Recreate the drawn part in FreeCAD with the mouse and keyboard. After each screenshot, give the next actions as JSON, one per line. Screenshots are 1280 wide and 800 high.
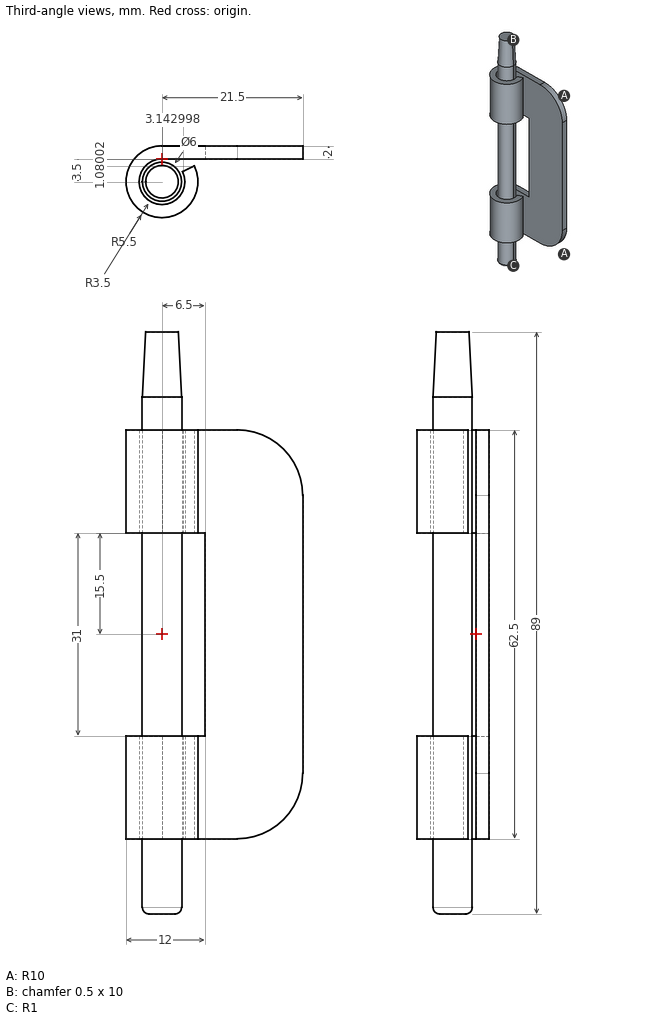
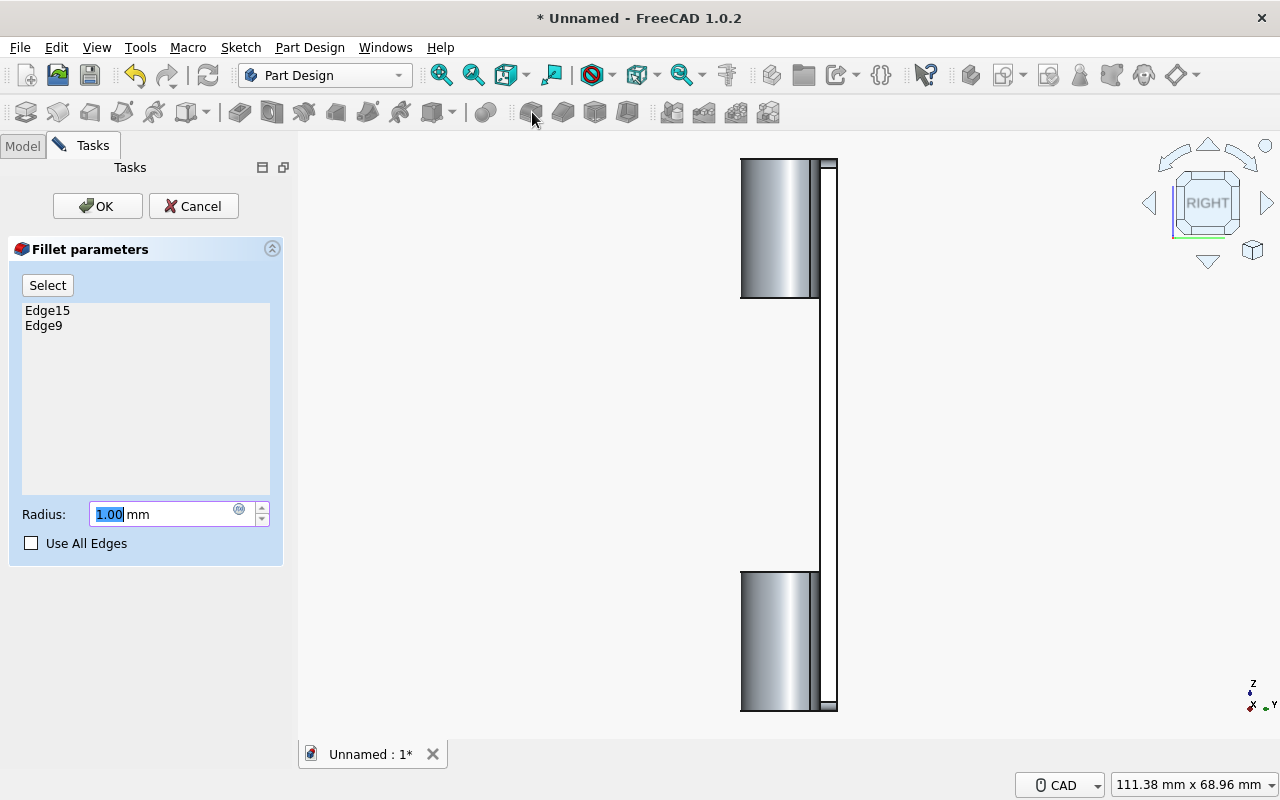
{"action": "type", "text": "10"}
{"action": "key", "text": "Tab"}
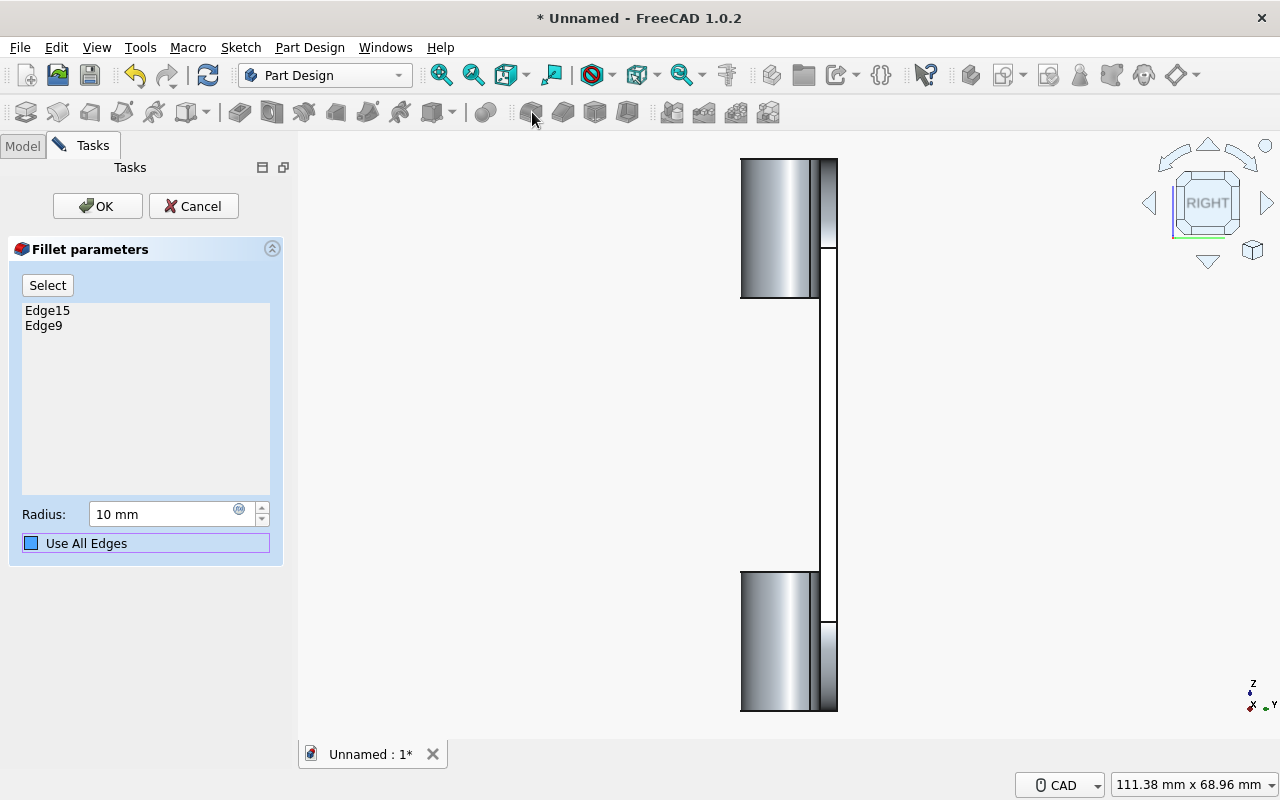
{"action": "left_click", "coordinate": [98, 206]}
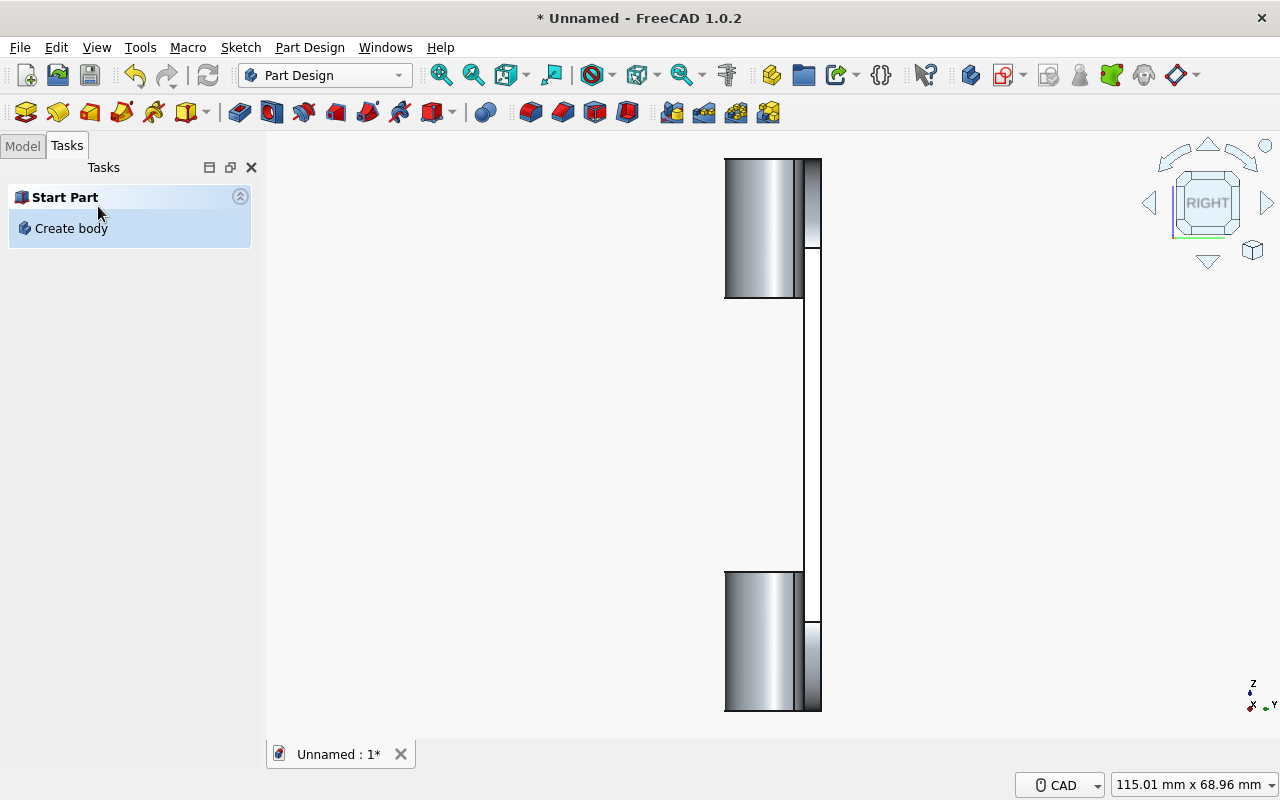
{"action": "left_click", "coordinate": [972, 76]}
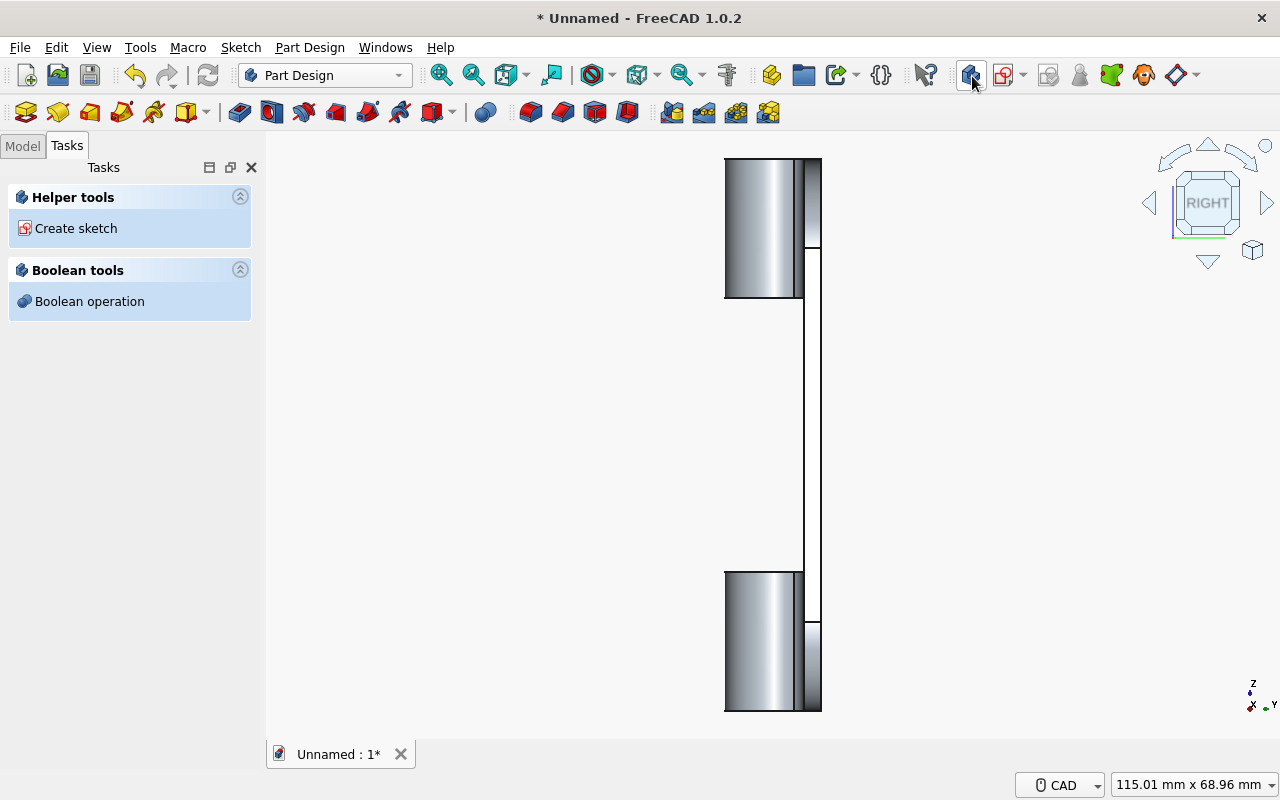
{"action": "left_click", "coordinate": [23, 145]}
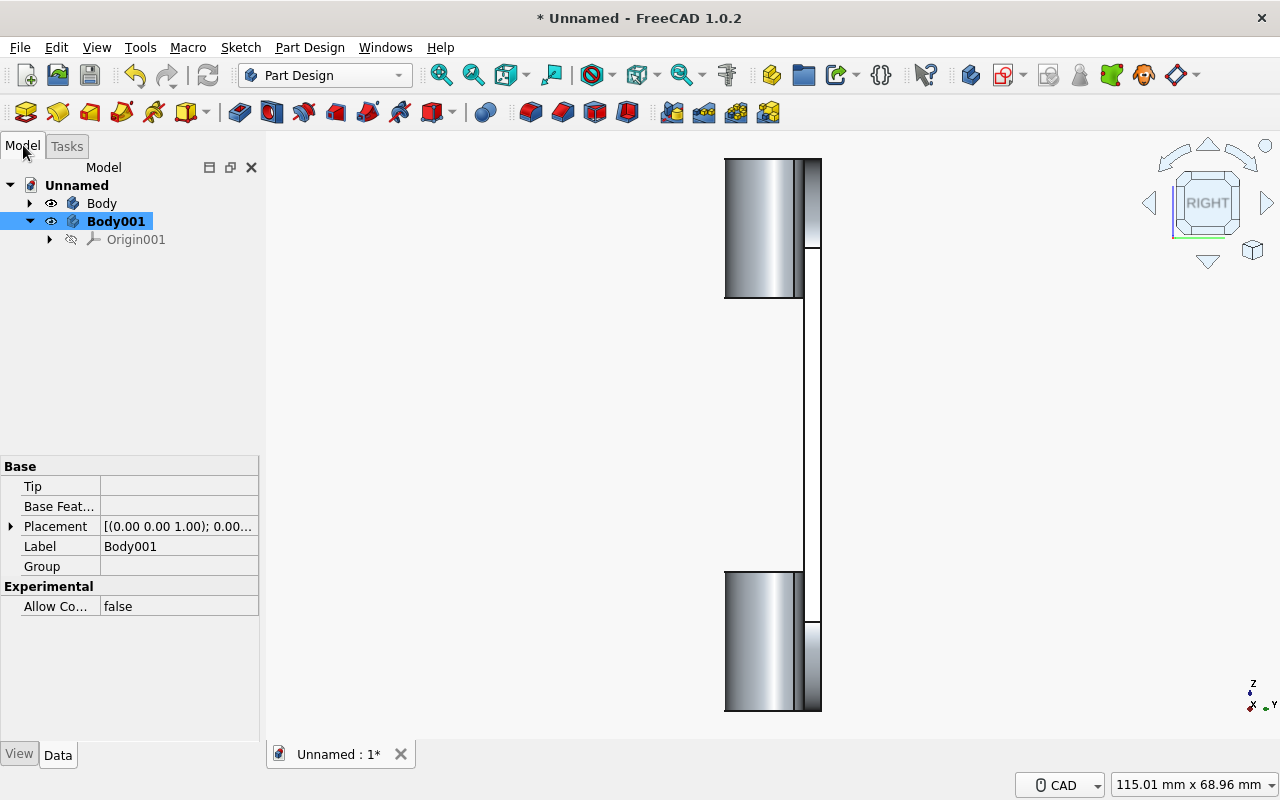
{"action": "left_click", "coordinate": [50, 239]}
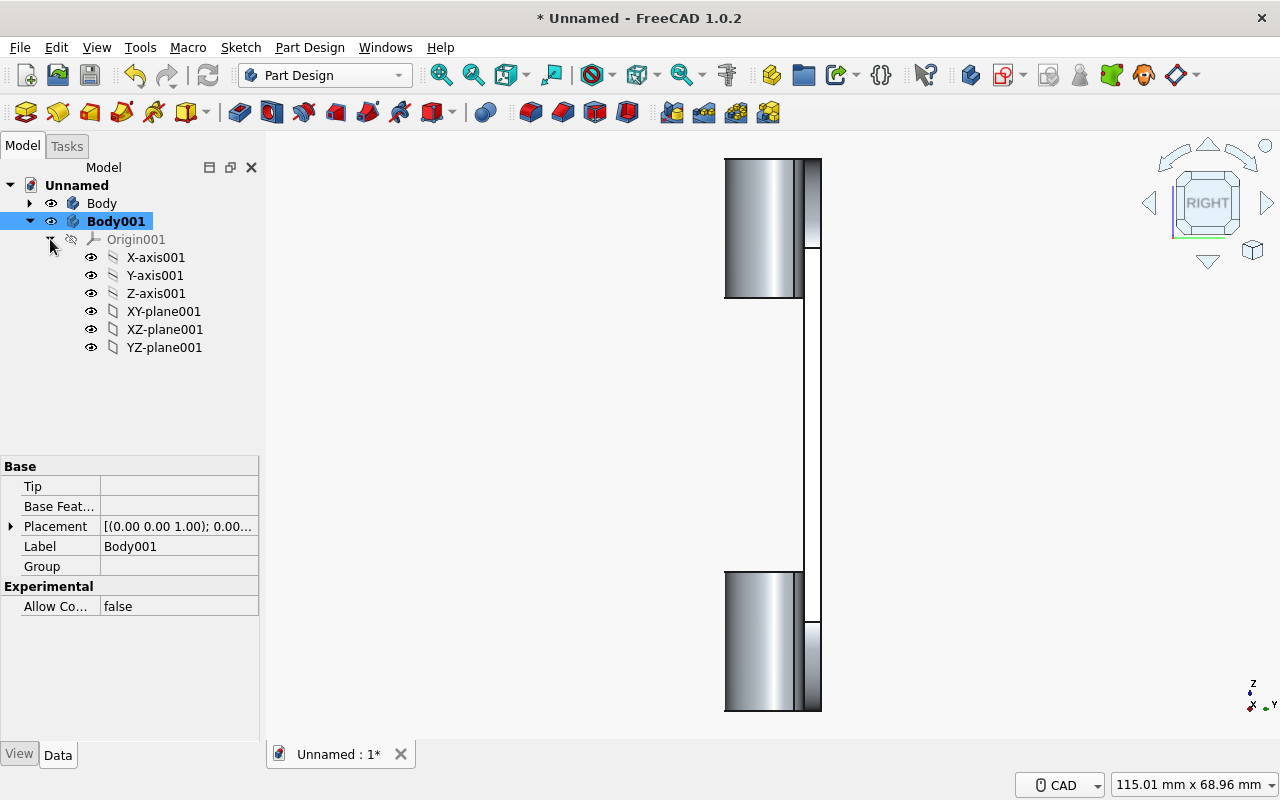
{"action": "left_click", "coordinate": [136, 311]}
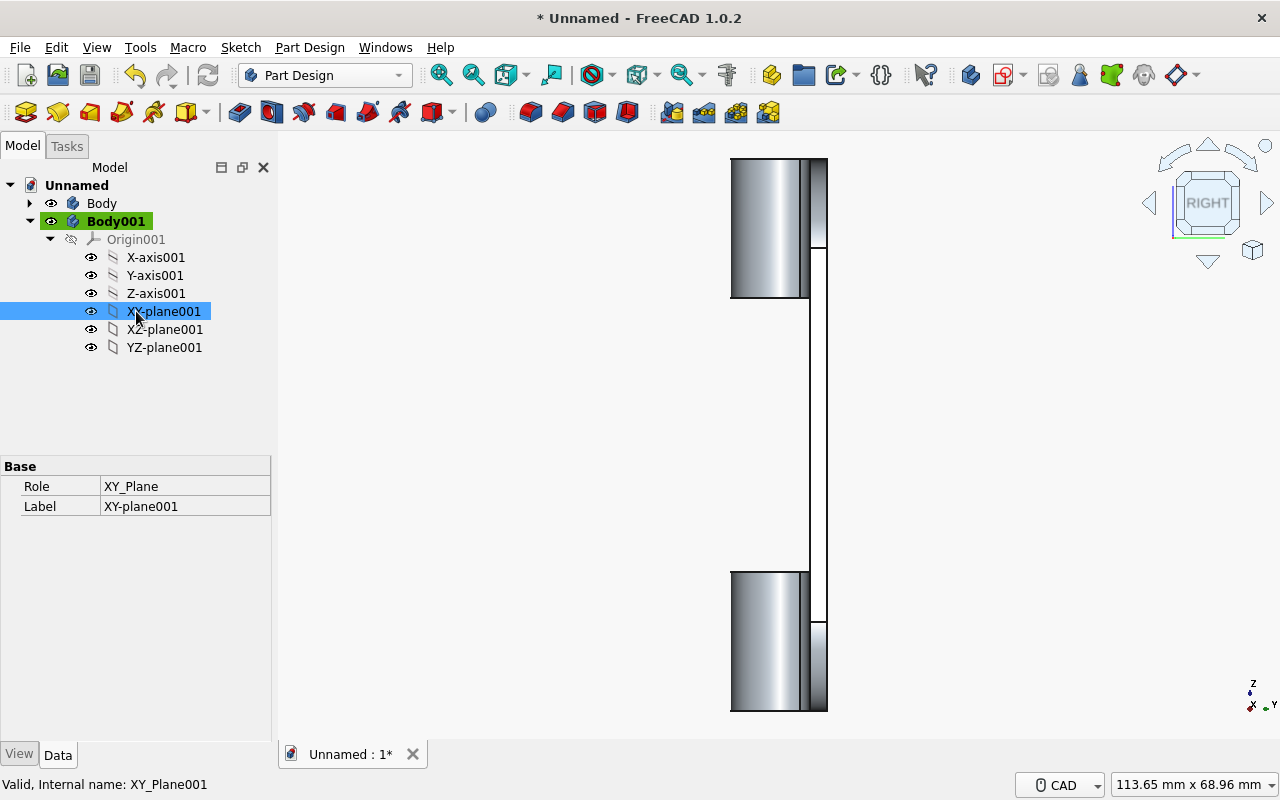
{"action": "left_click", "coordinate": [1176, 76]}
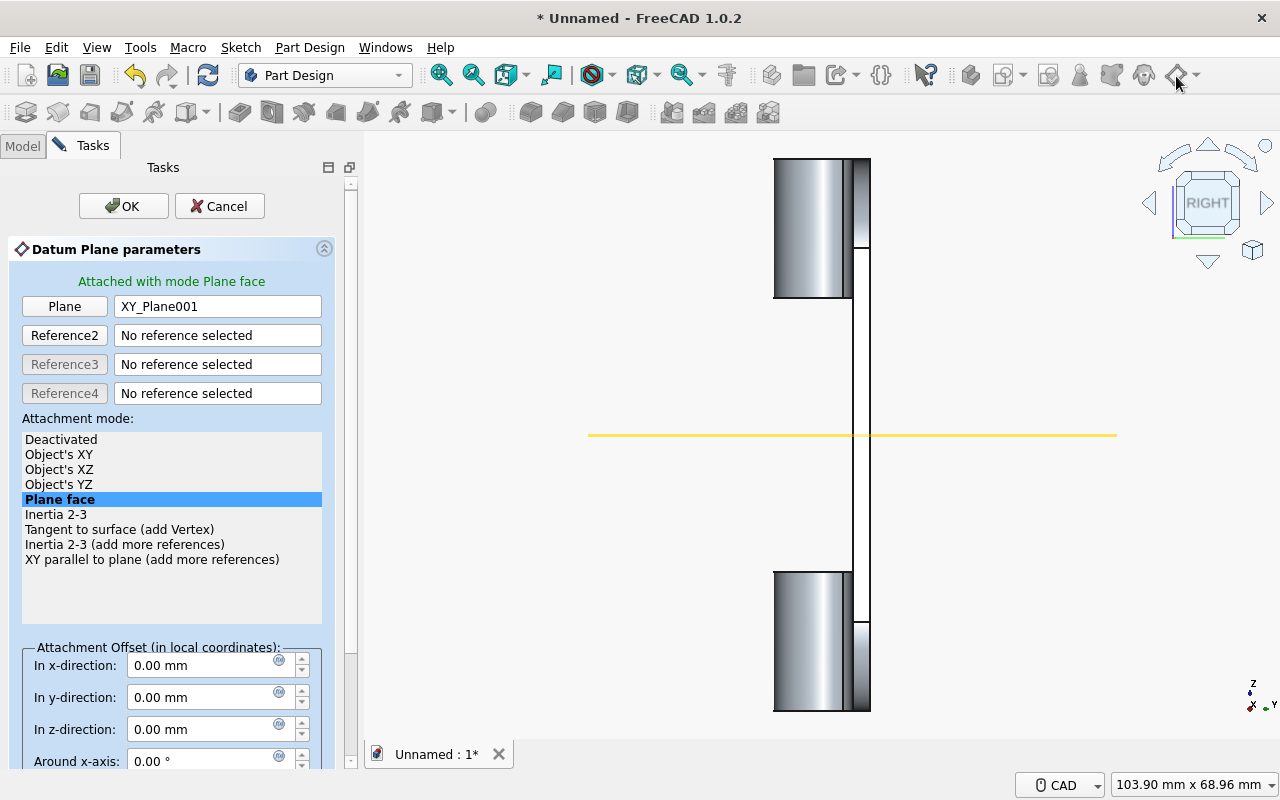
{"action": "triple_click", "coordinate": [210, 729]}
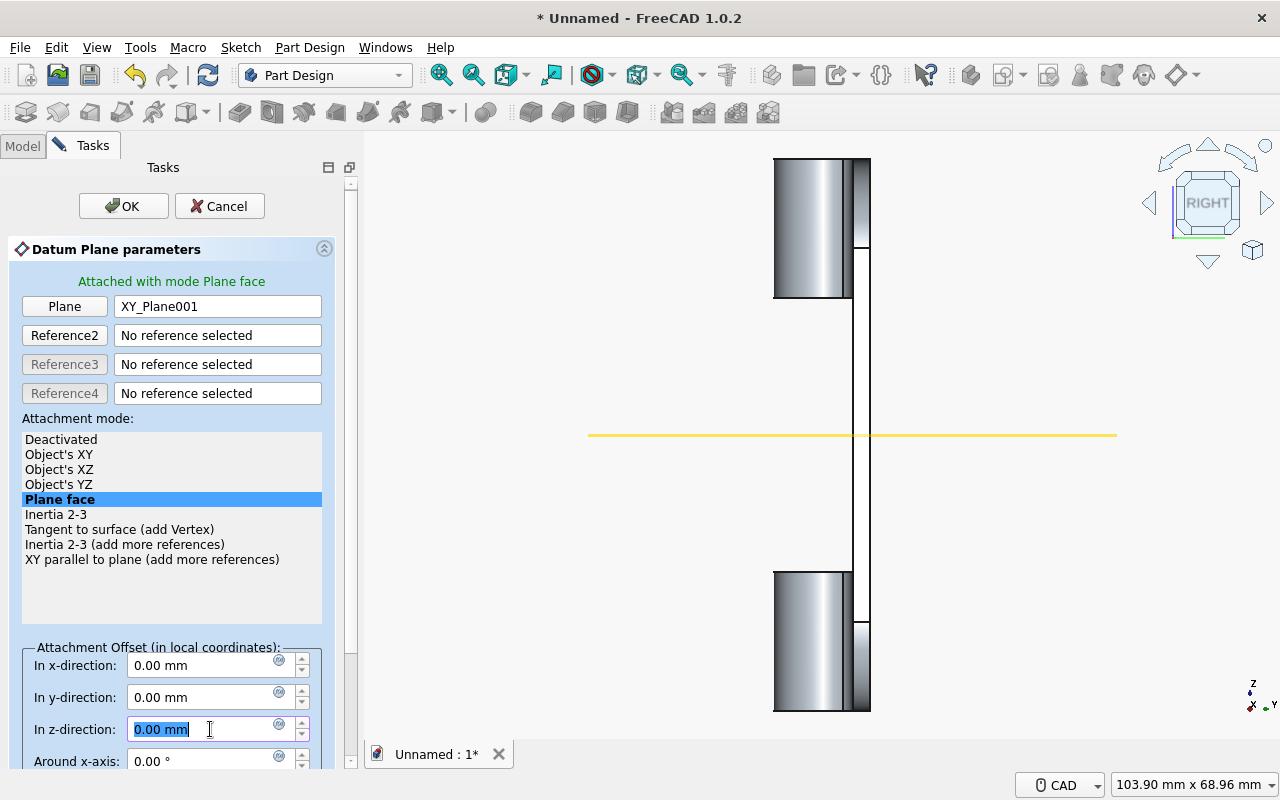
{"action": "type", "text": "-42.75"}
{"action": "key", "text": "Tab"}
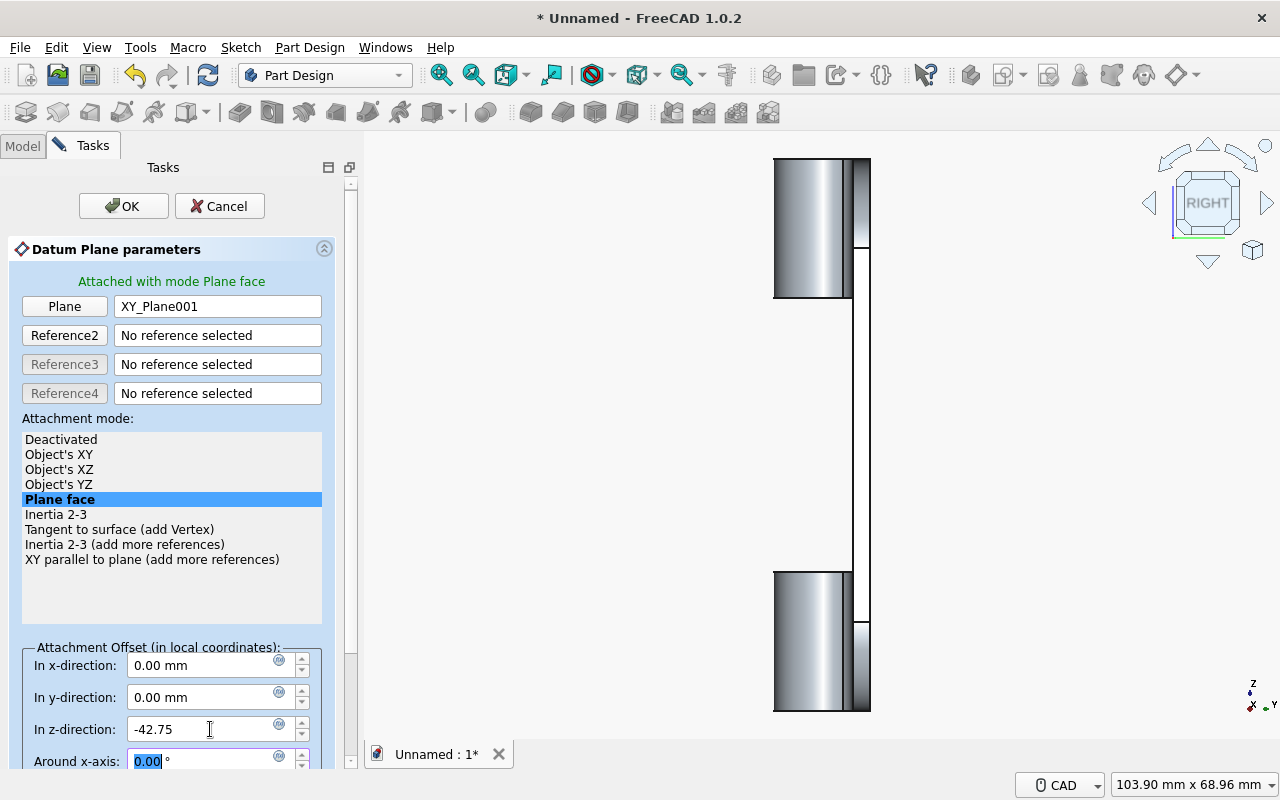
{"action": "left_click", "coordinate": [124, 206]}